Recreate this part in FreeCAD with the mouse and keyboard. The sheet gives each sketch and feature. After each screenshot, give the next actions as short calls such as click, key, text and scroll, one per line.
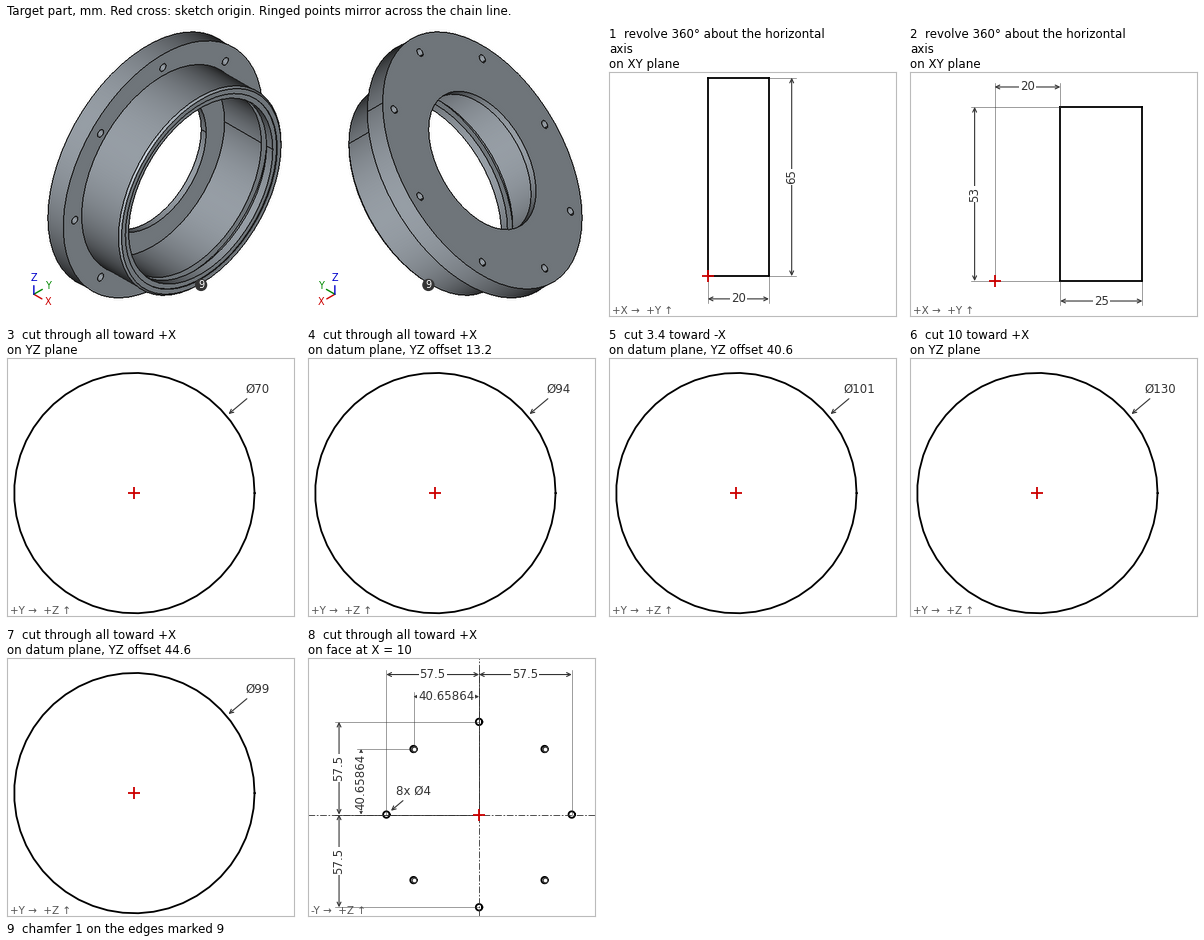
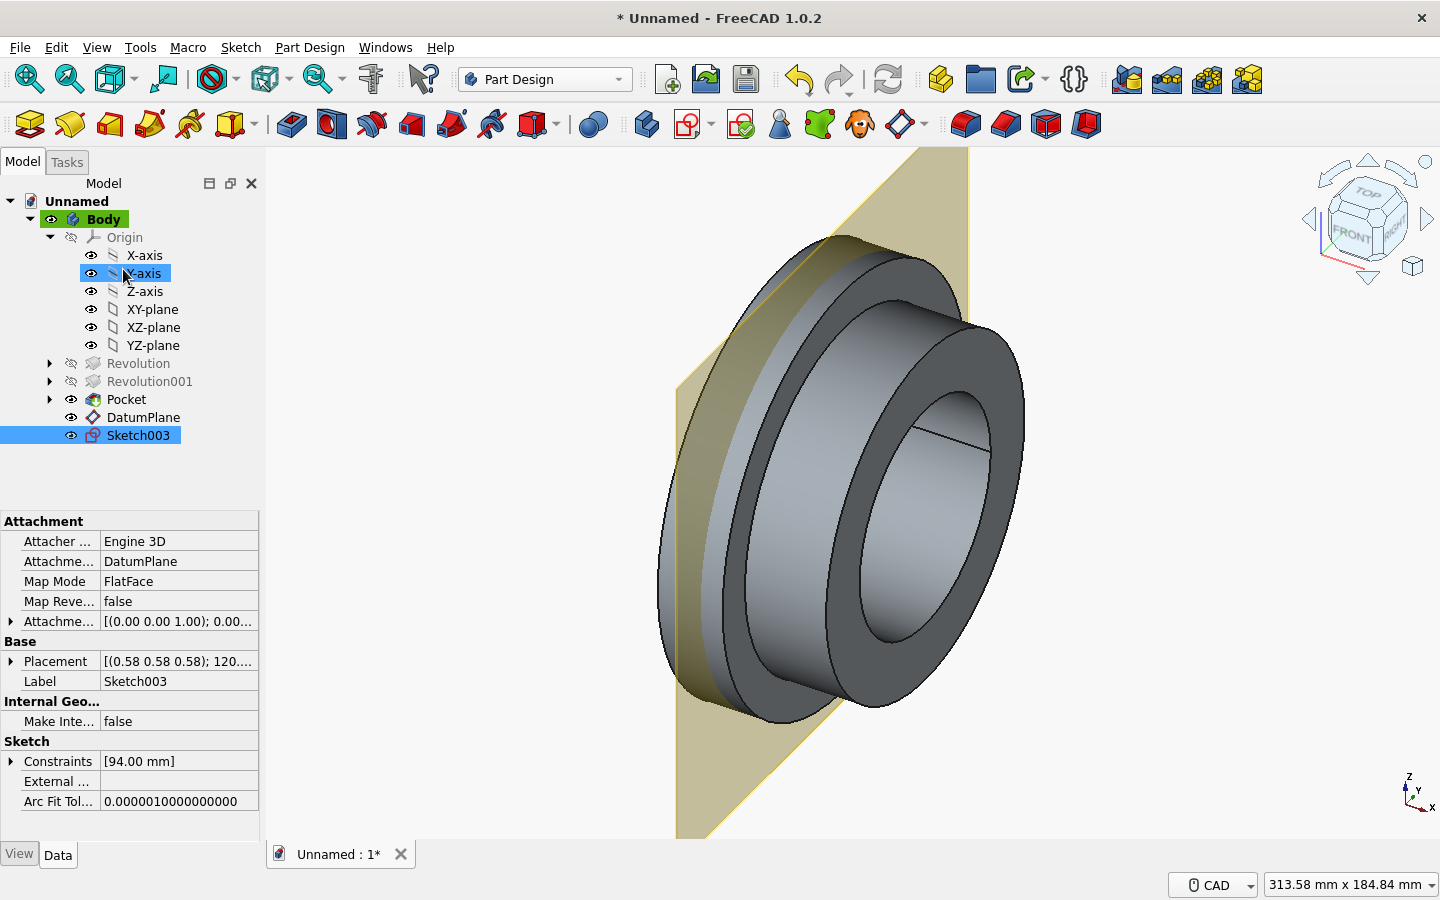
click(292, 124)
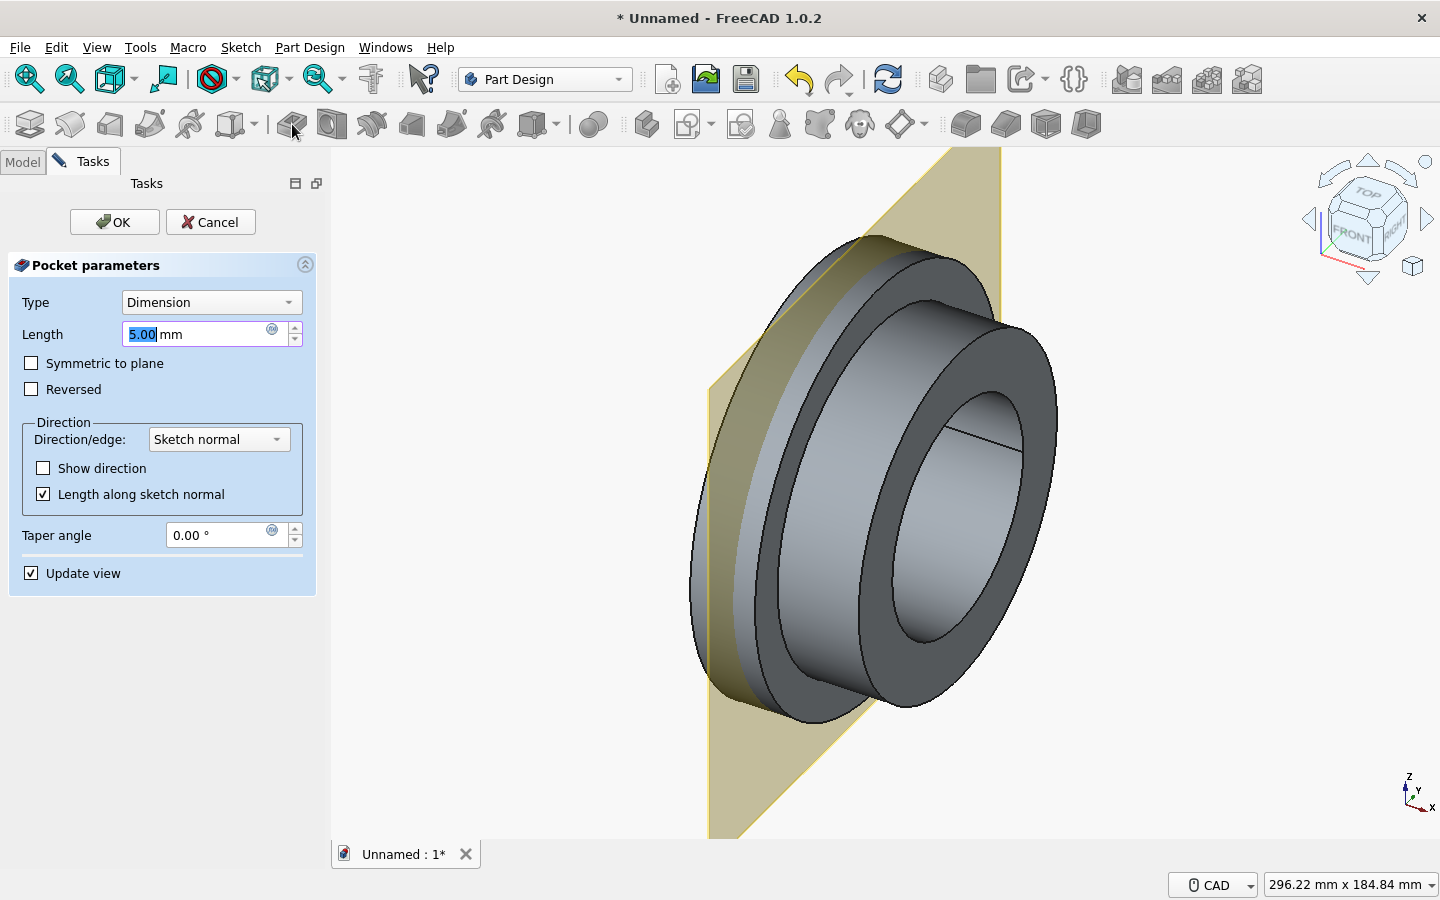
click(212, 302)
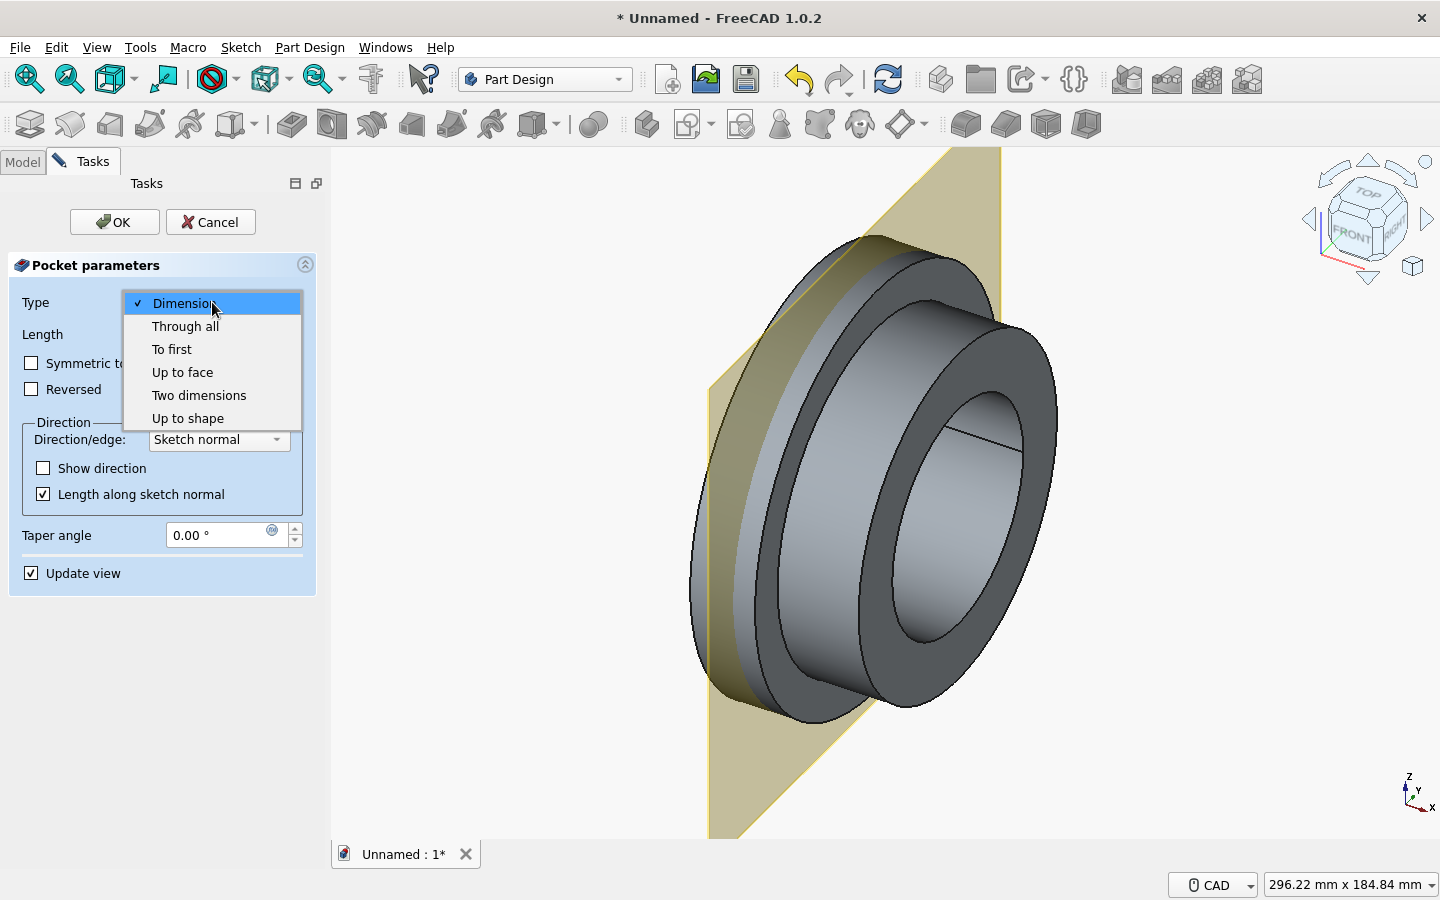
click(212, 326)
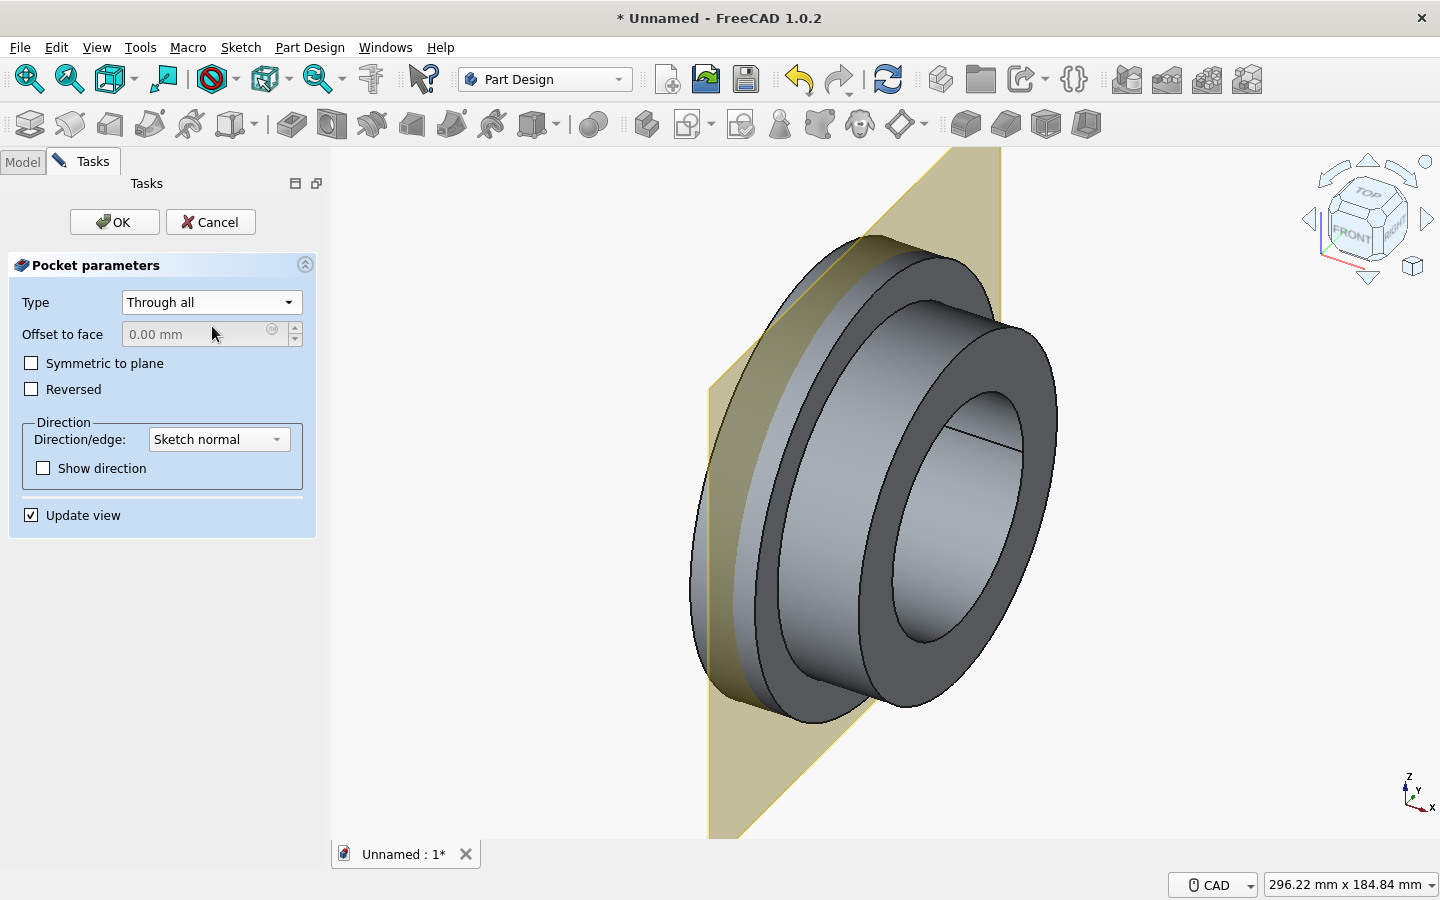
click(30, 389)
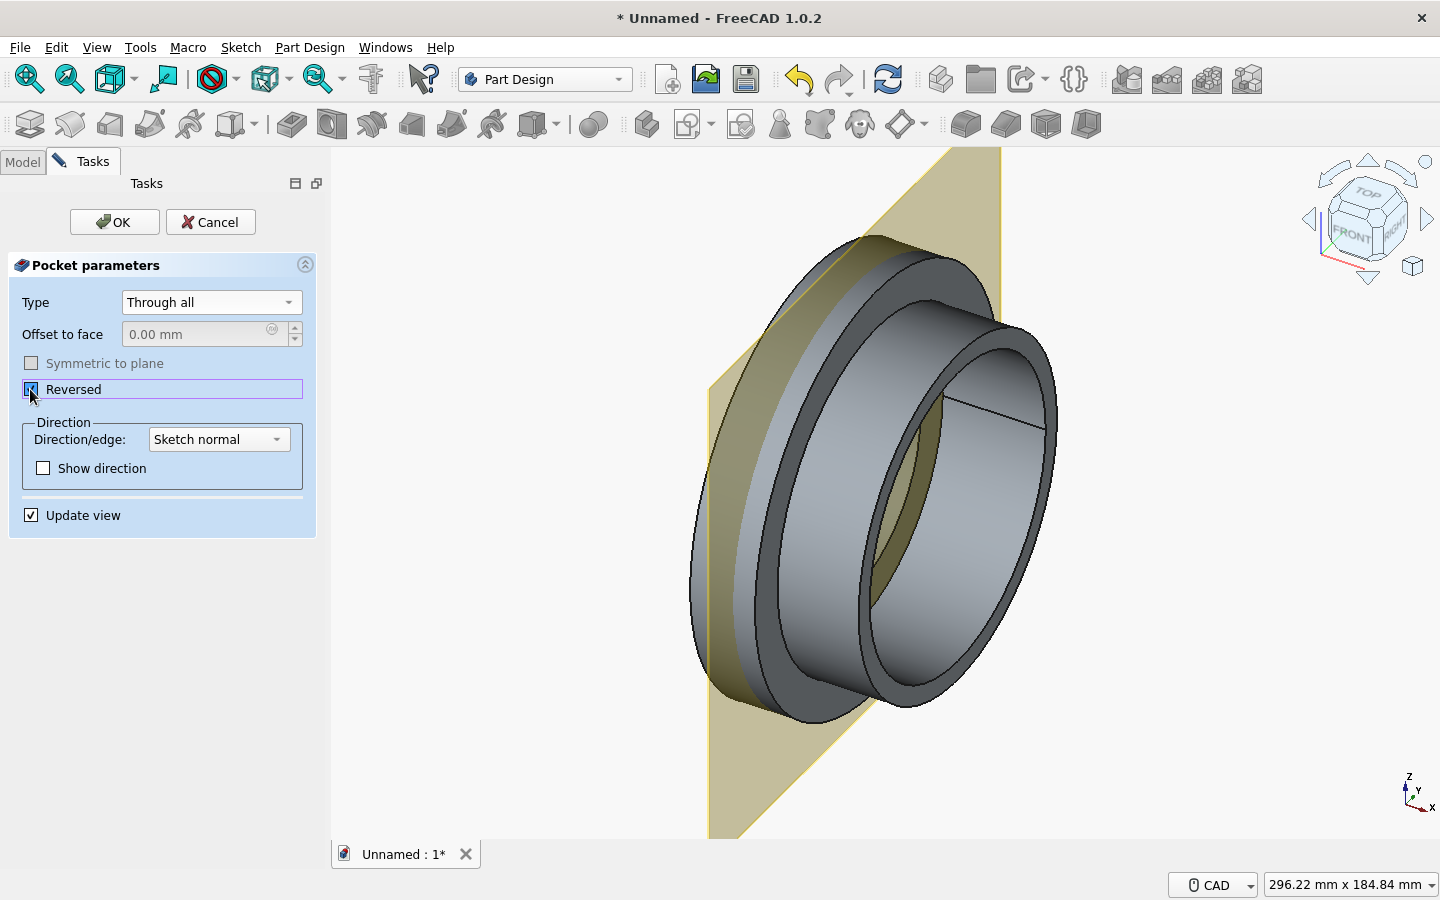
click(115, 222)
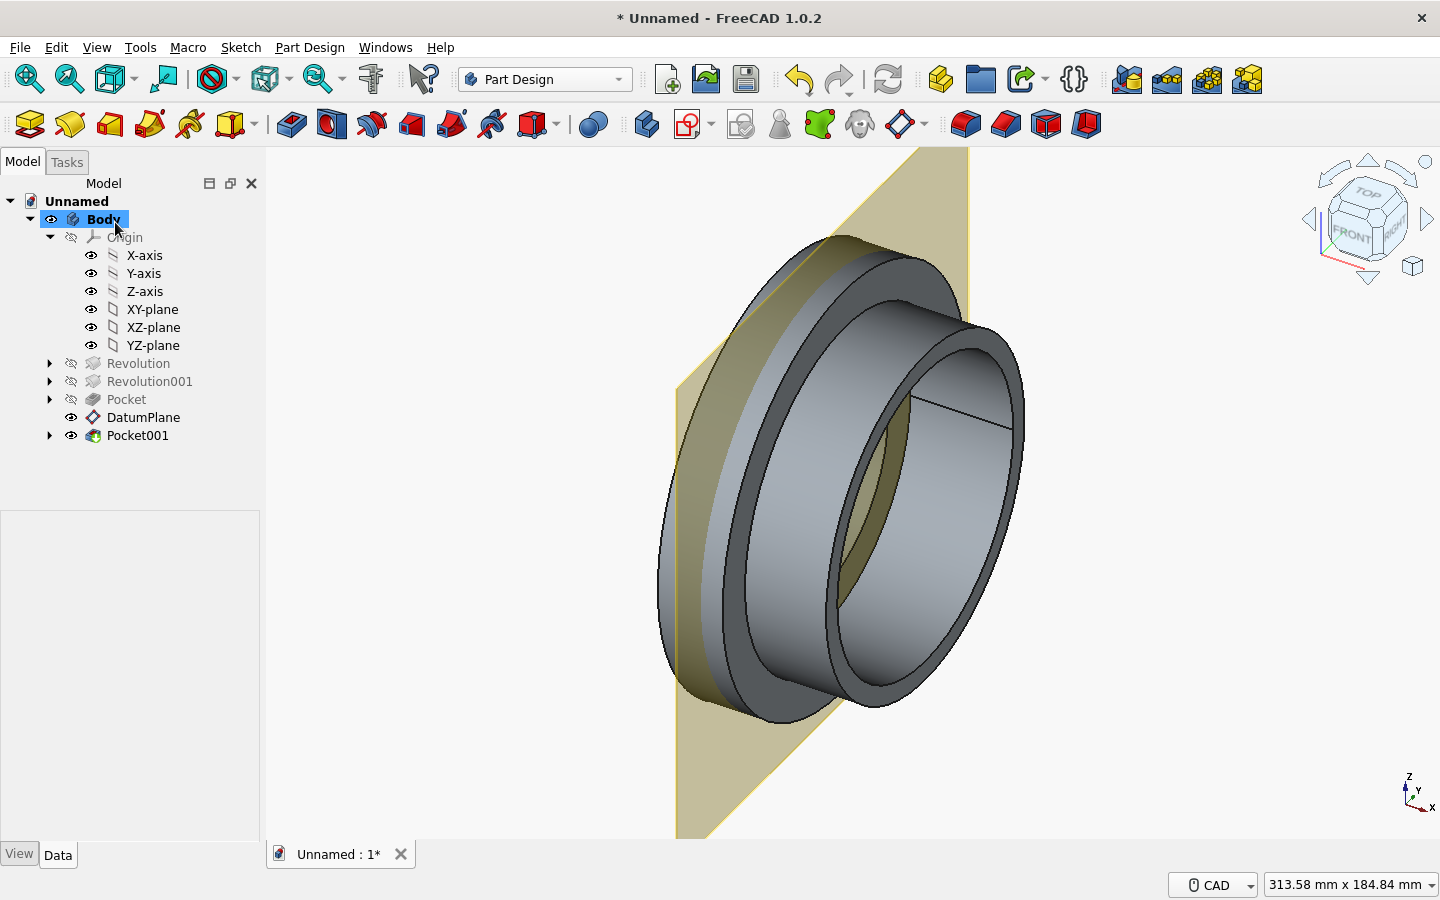
click(116, 417)
key(space)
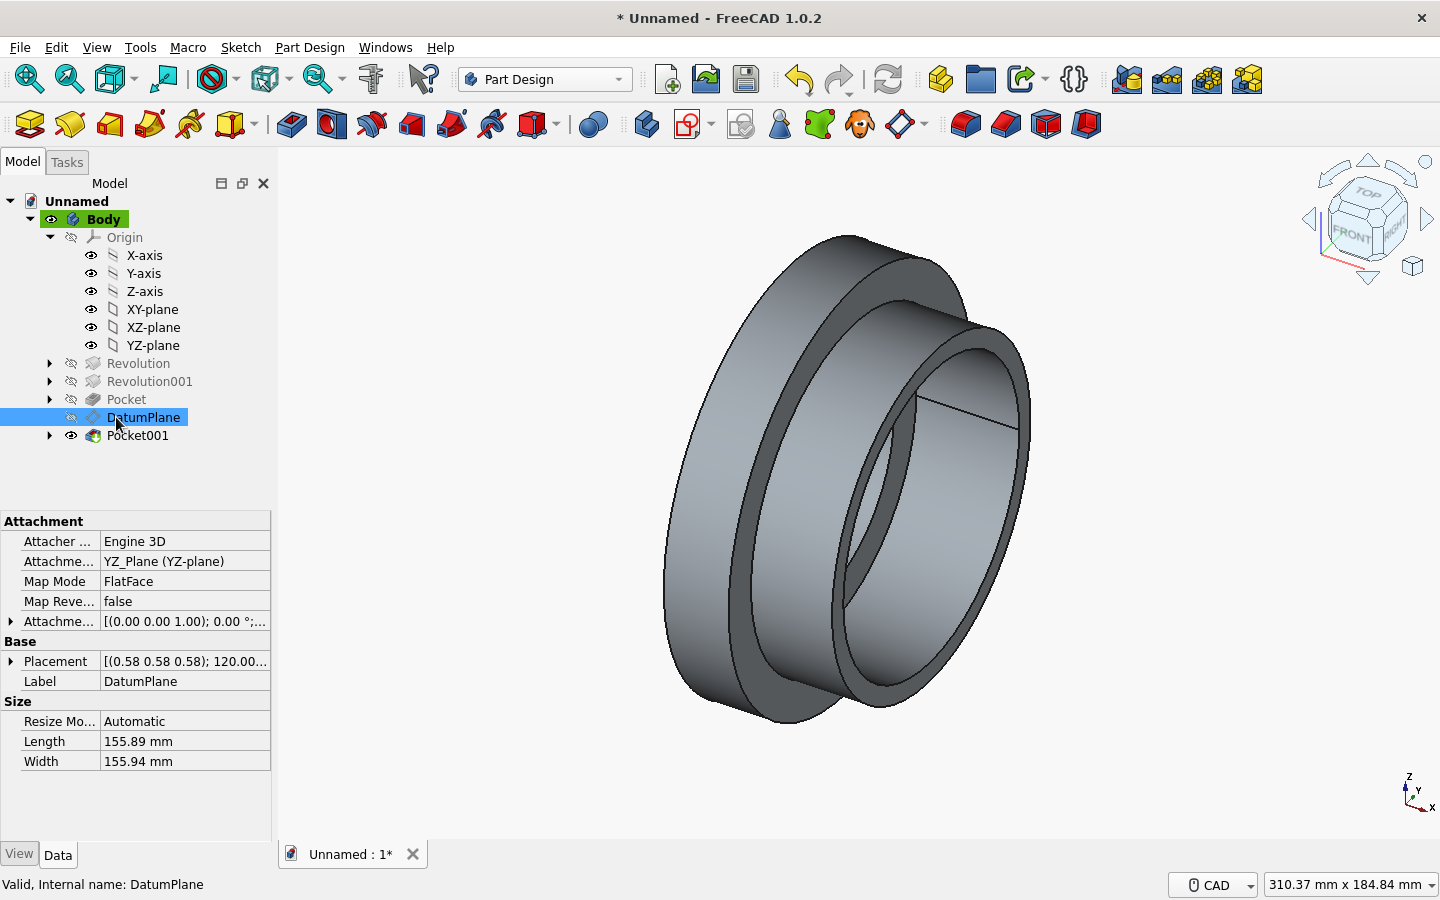
click(136, 345)